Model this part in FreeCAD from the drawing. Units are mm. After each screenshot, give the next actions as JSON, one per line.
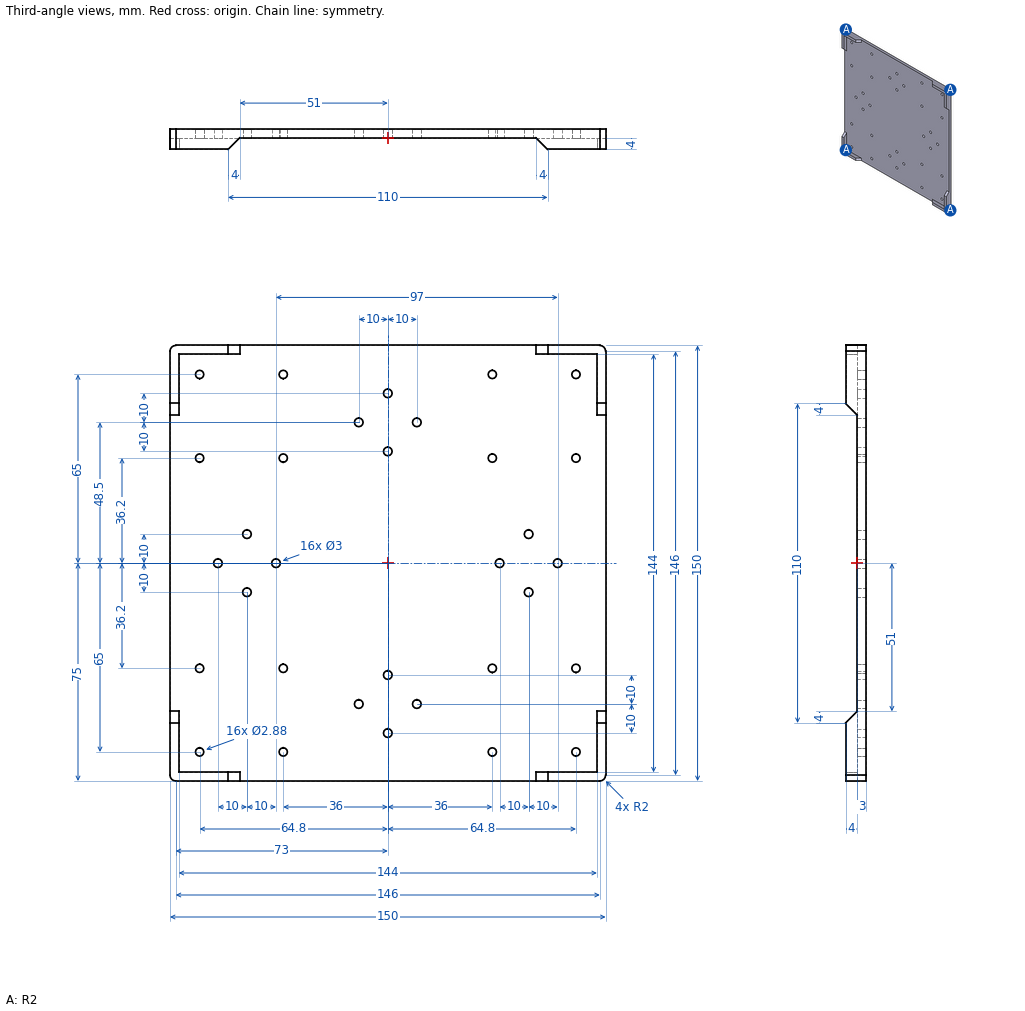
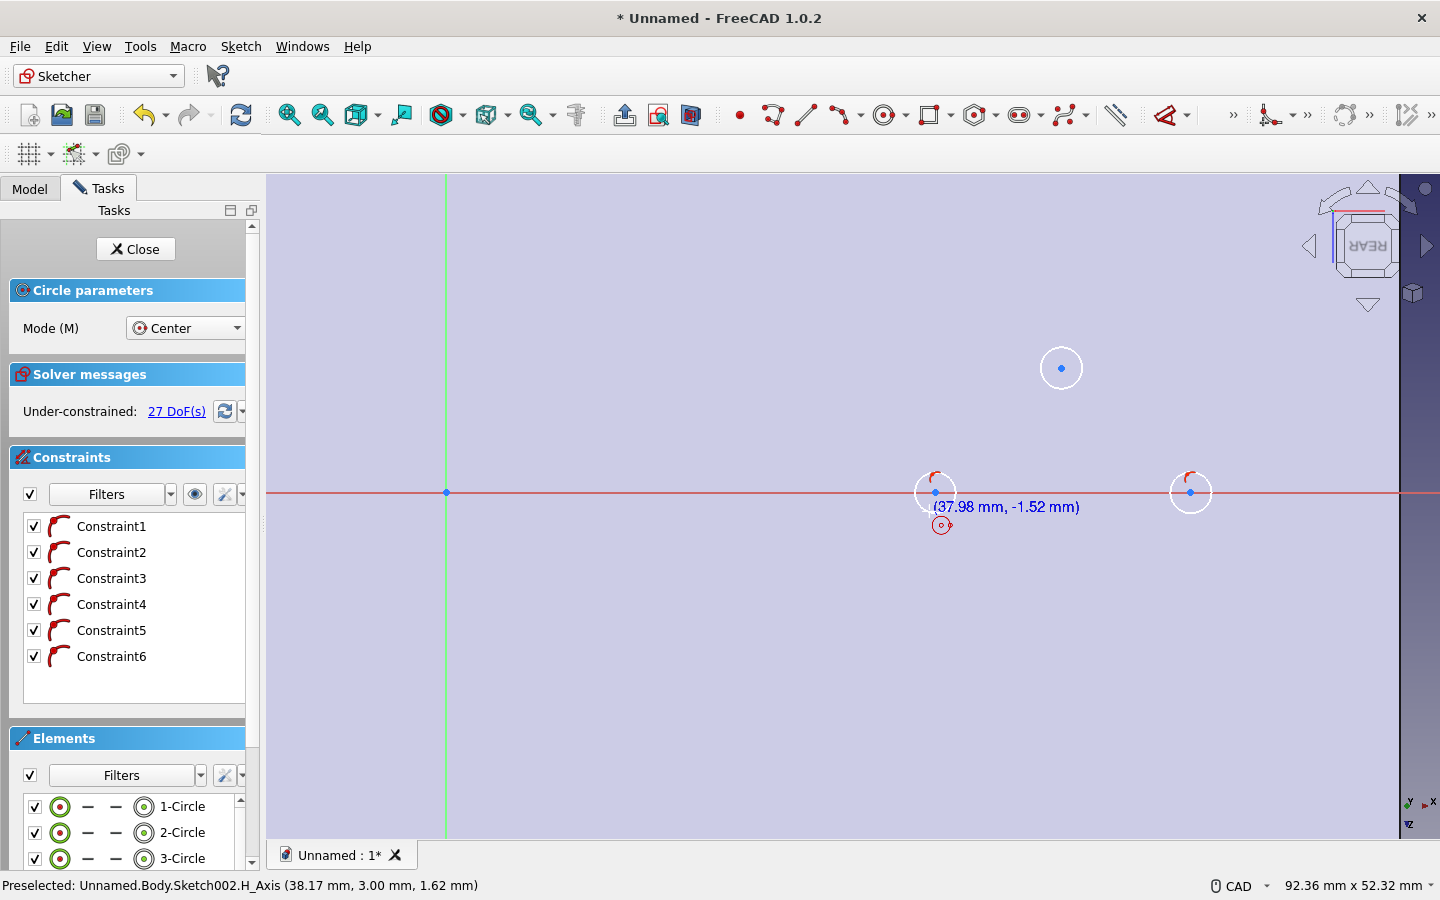
{"action": "scroll", "coordinate": [930, 512], "scroll_direction": "down", "scroll_amount": 6}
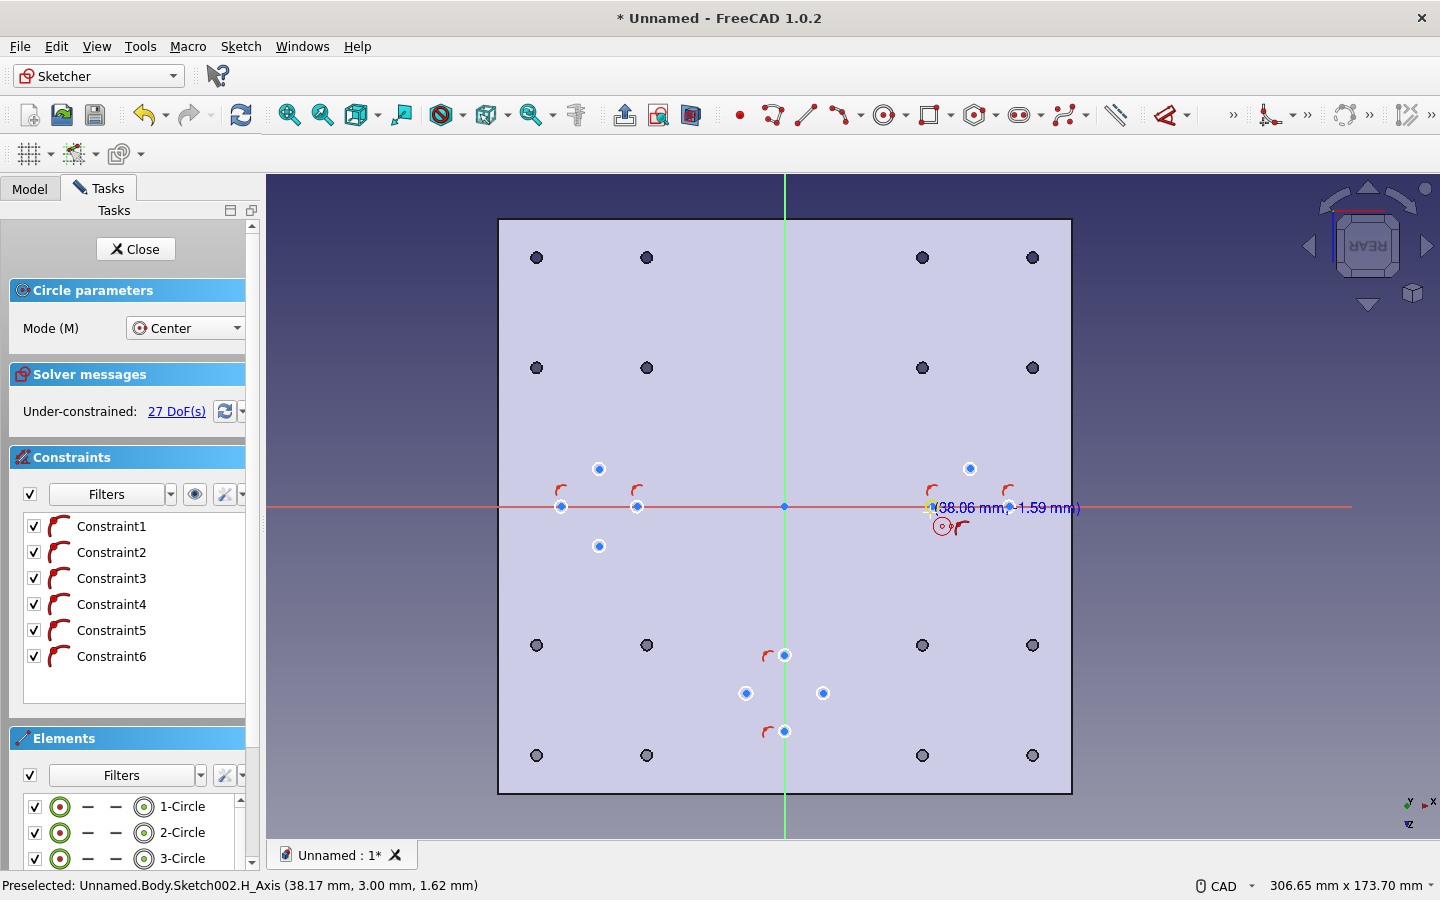
{"action": "scroll", "coordinate": [785, 359], "scroll_direction": "up", "scroll_amount": 7}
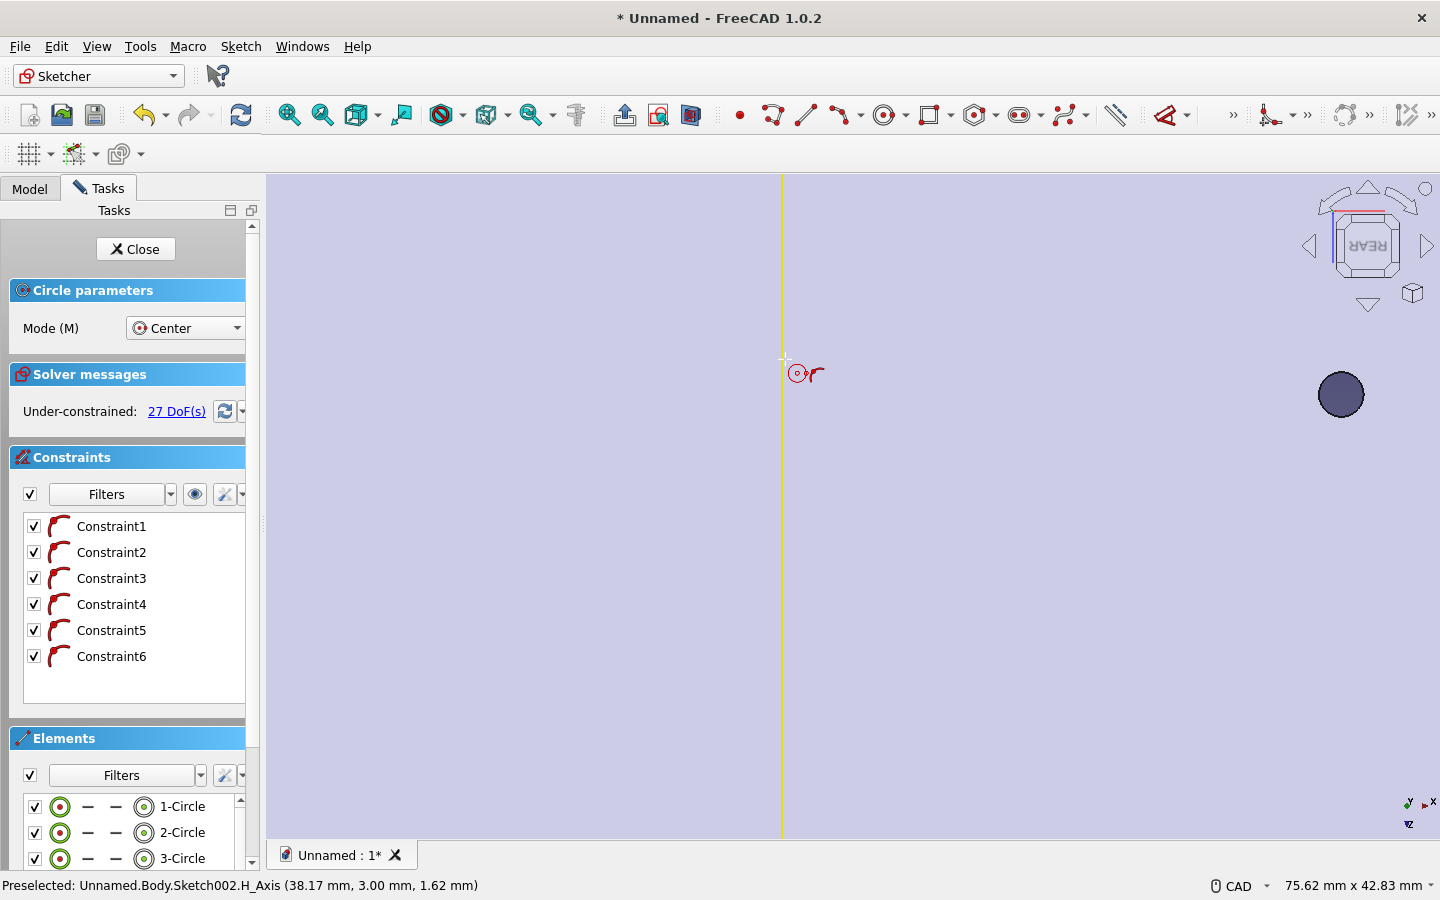
{"action": "scroll", "coordinate": [785, 359], "scroll_direction": "down", "scroll_amount": 7}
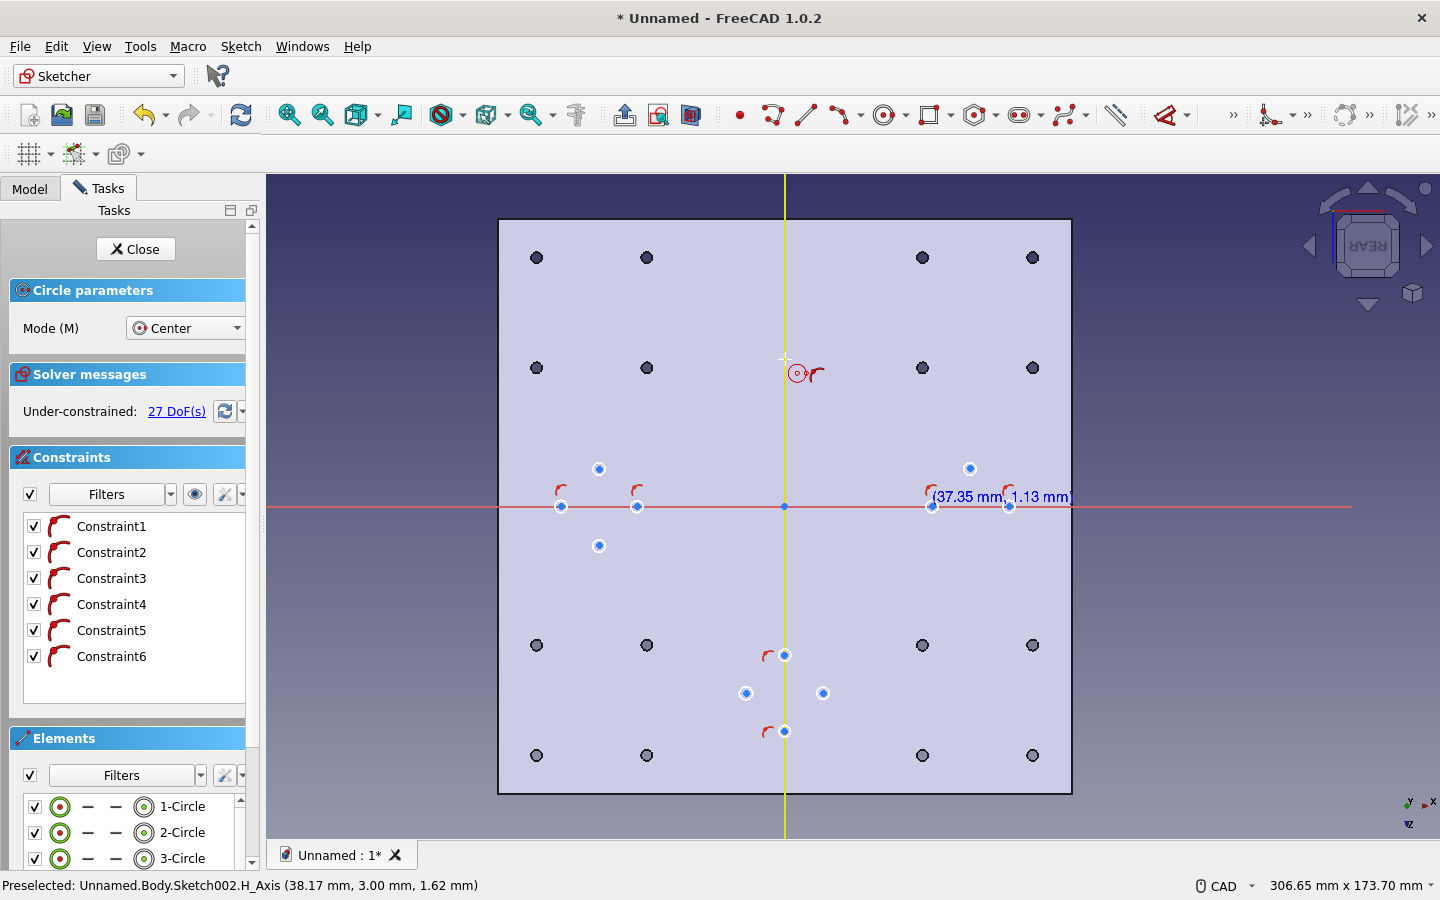
{"action": "left_click", "coordinate": [785, 359]}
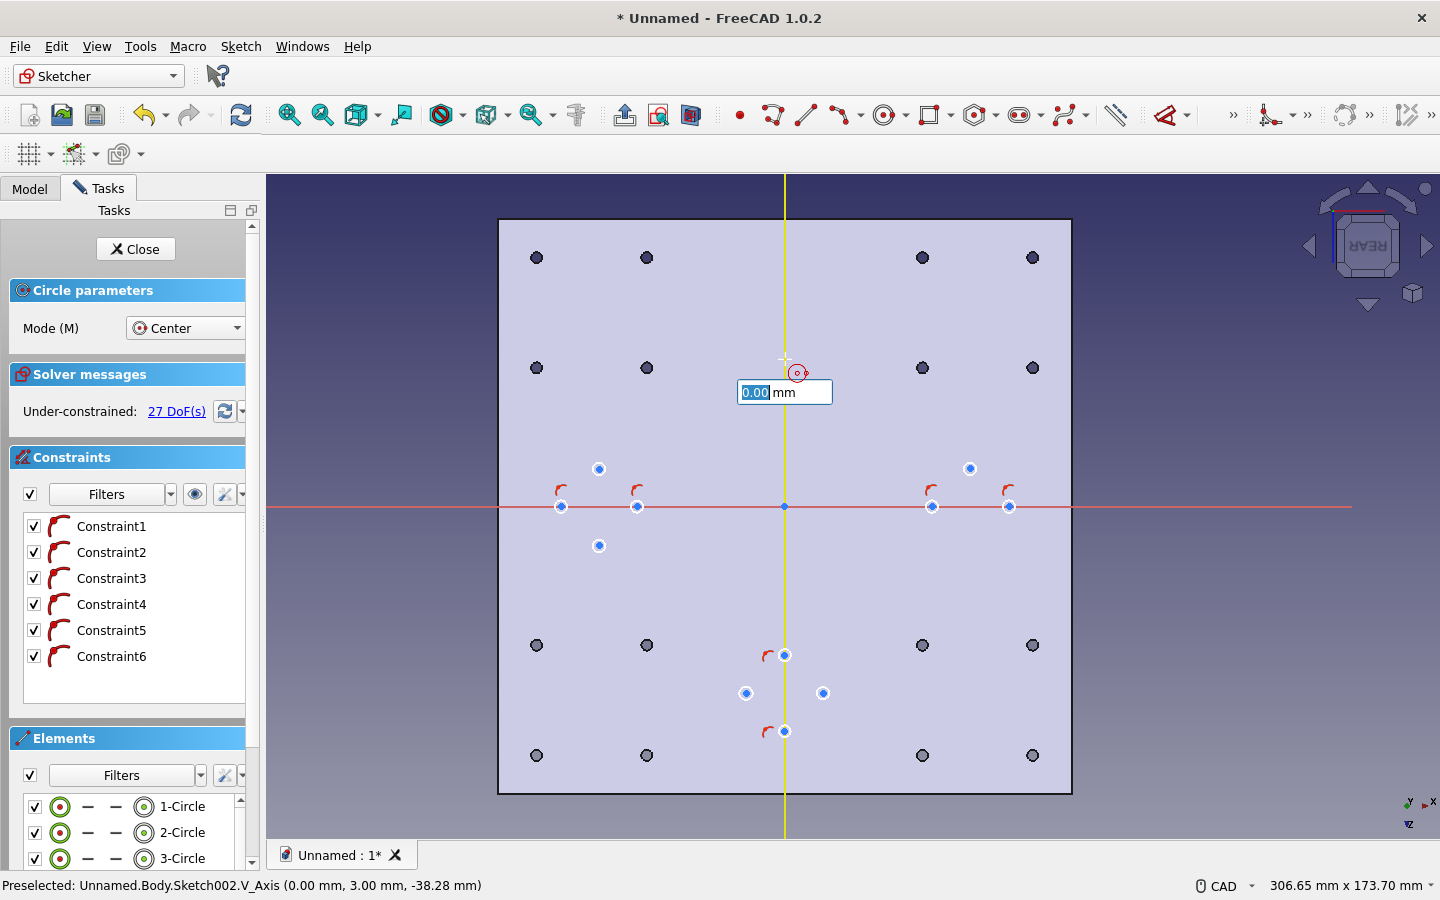
{"action": "scroll", "coordinate": [790, 357], "scroll_direction": "up", "scroll_amount": 6}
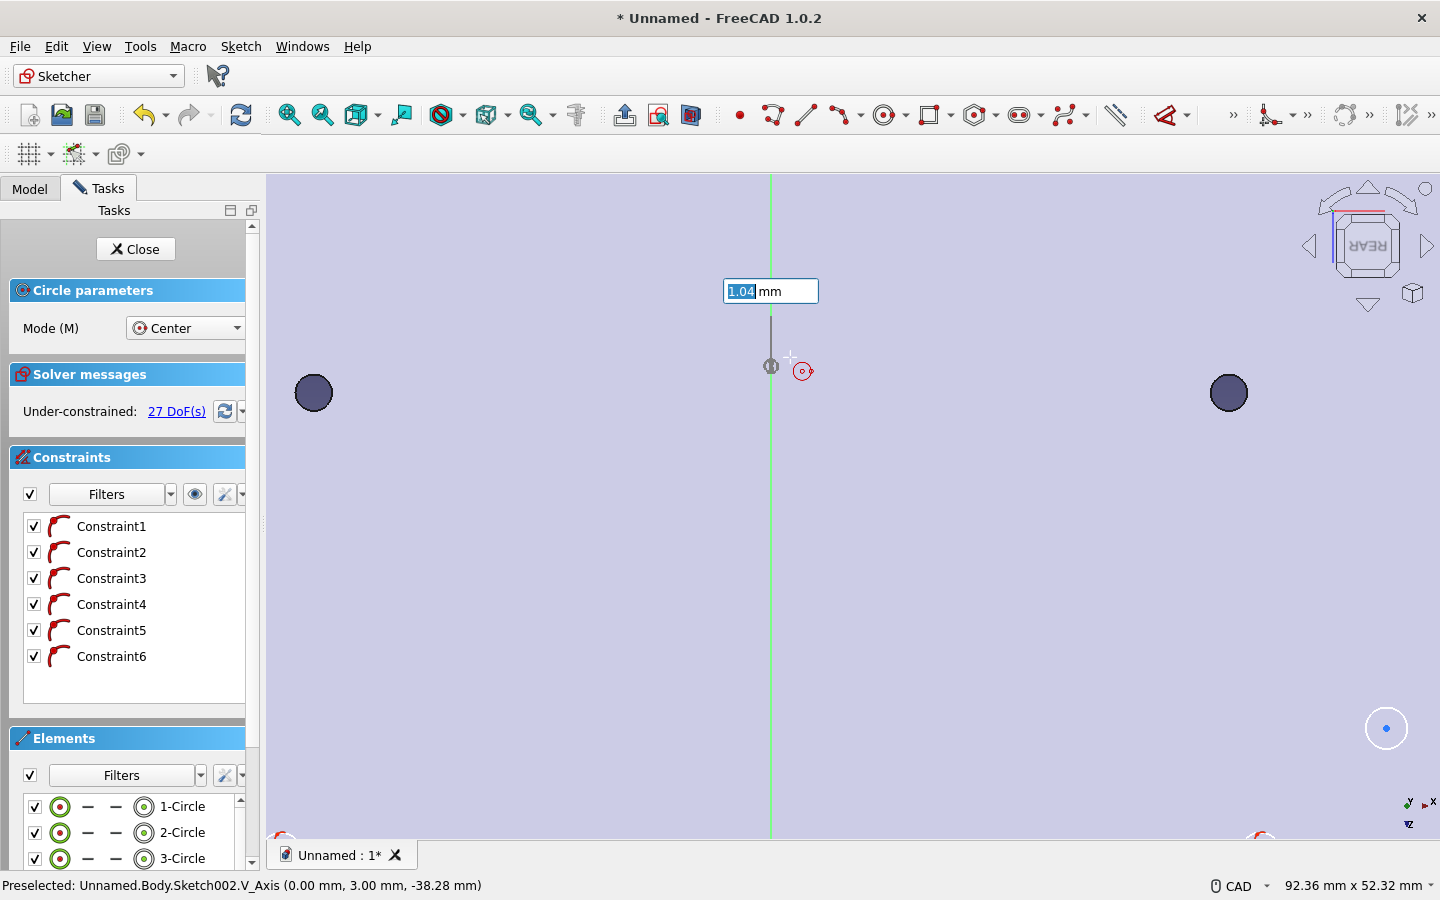
{"action": "left_click", "coordinate": [789, 357]}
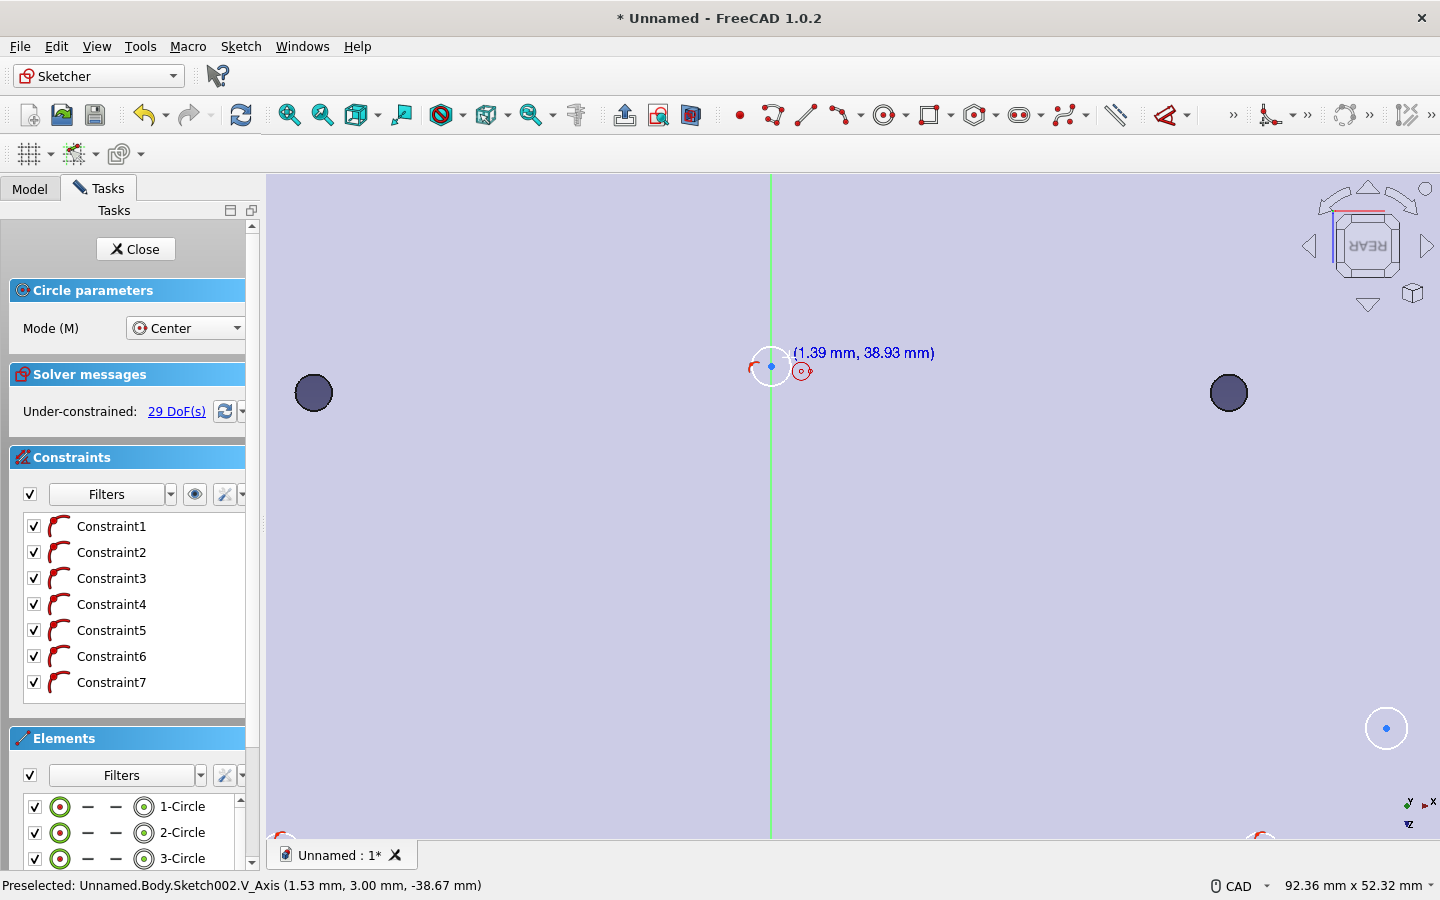
{"action": "scroll", "coordinate": [790, 357], "scroll_direction": "down", "scroll_amount": 6}